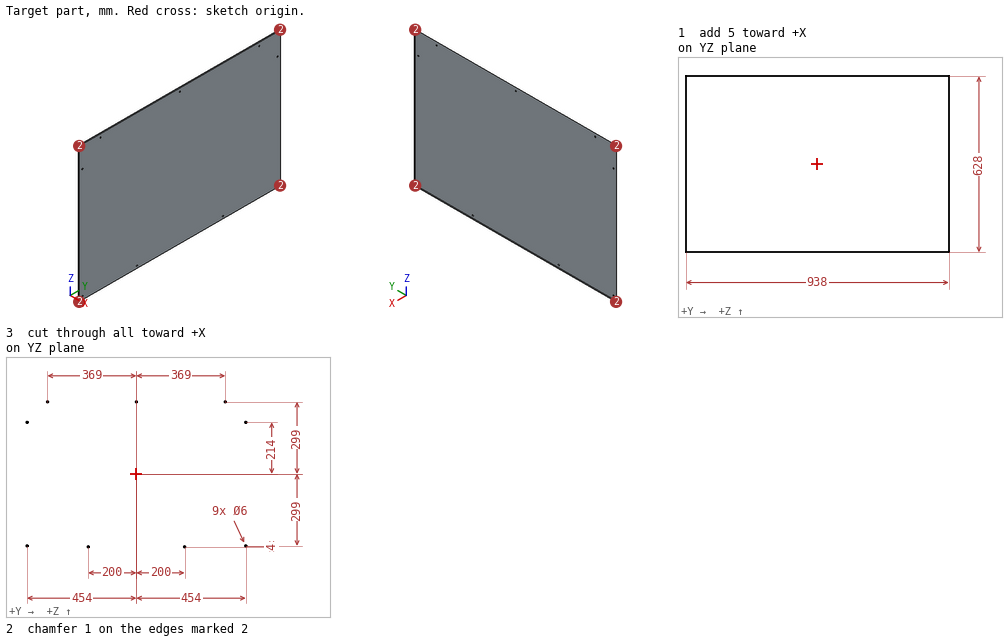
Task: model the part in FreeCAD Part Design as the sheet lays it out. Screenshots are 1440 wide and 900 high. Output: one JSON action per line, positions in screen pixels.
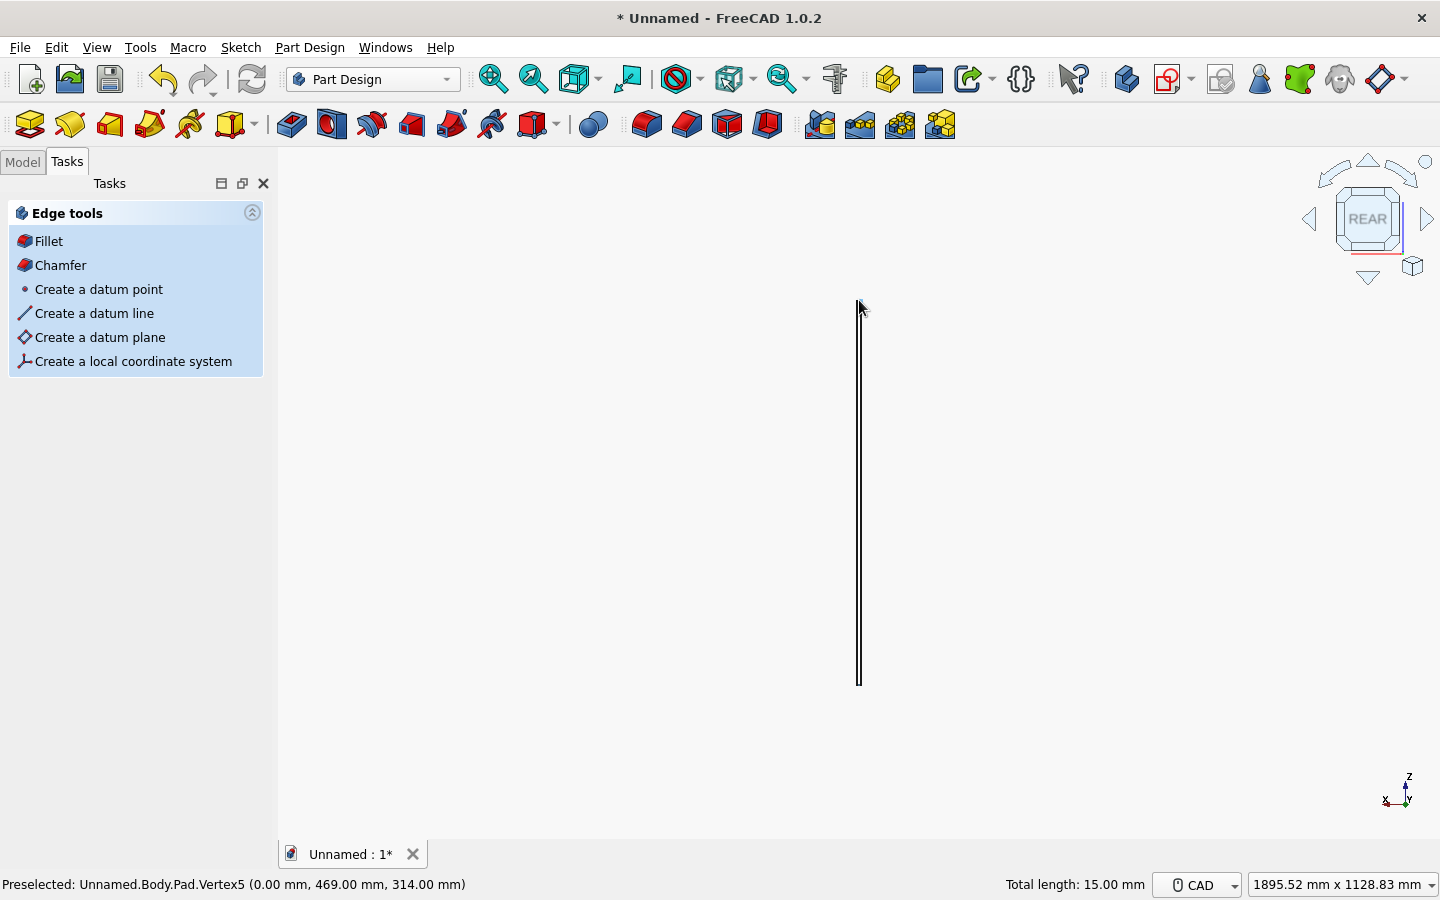
{"action": "key", "text": "6"}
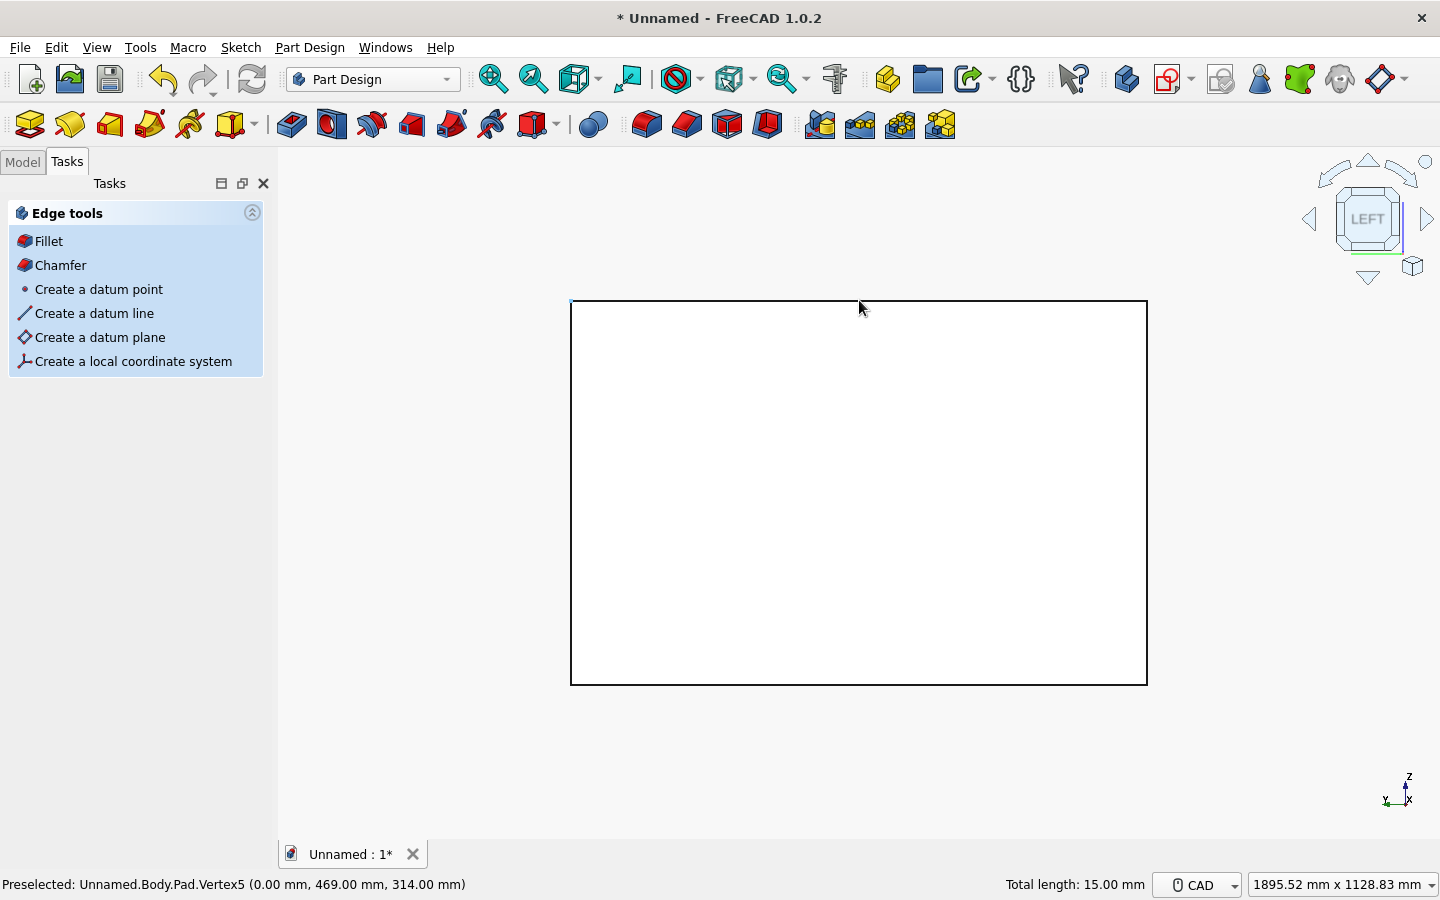
{"action": "scroll", "coordinate": [1147, 300], "scroll_direction": "up", "scroll_amount": 13}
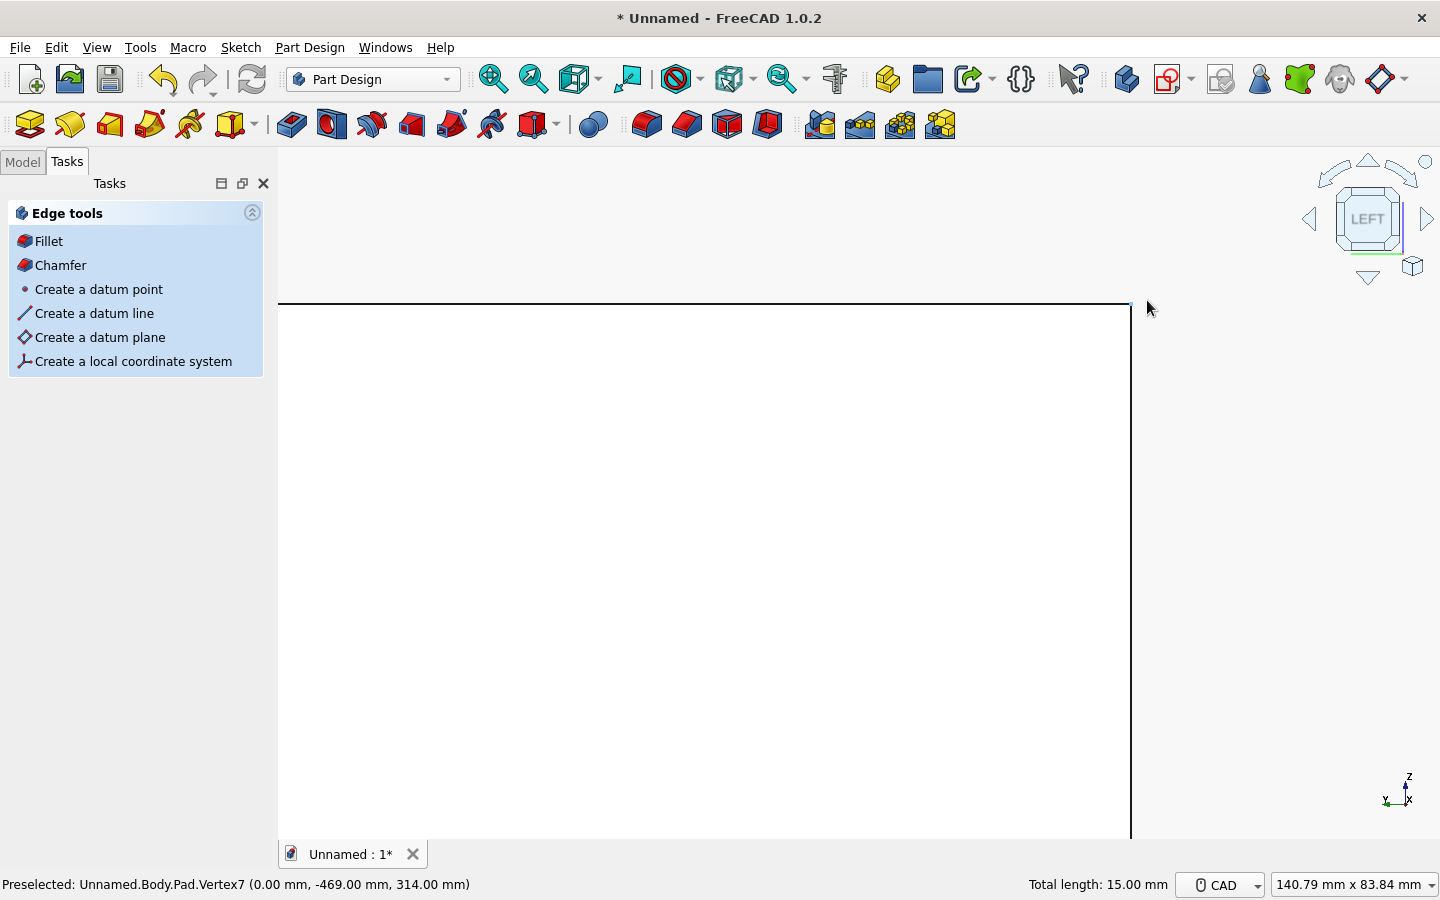
{"action": "key", "text": "v f"}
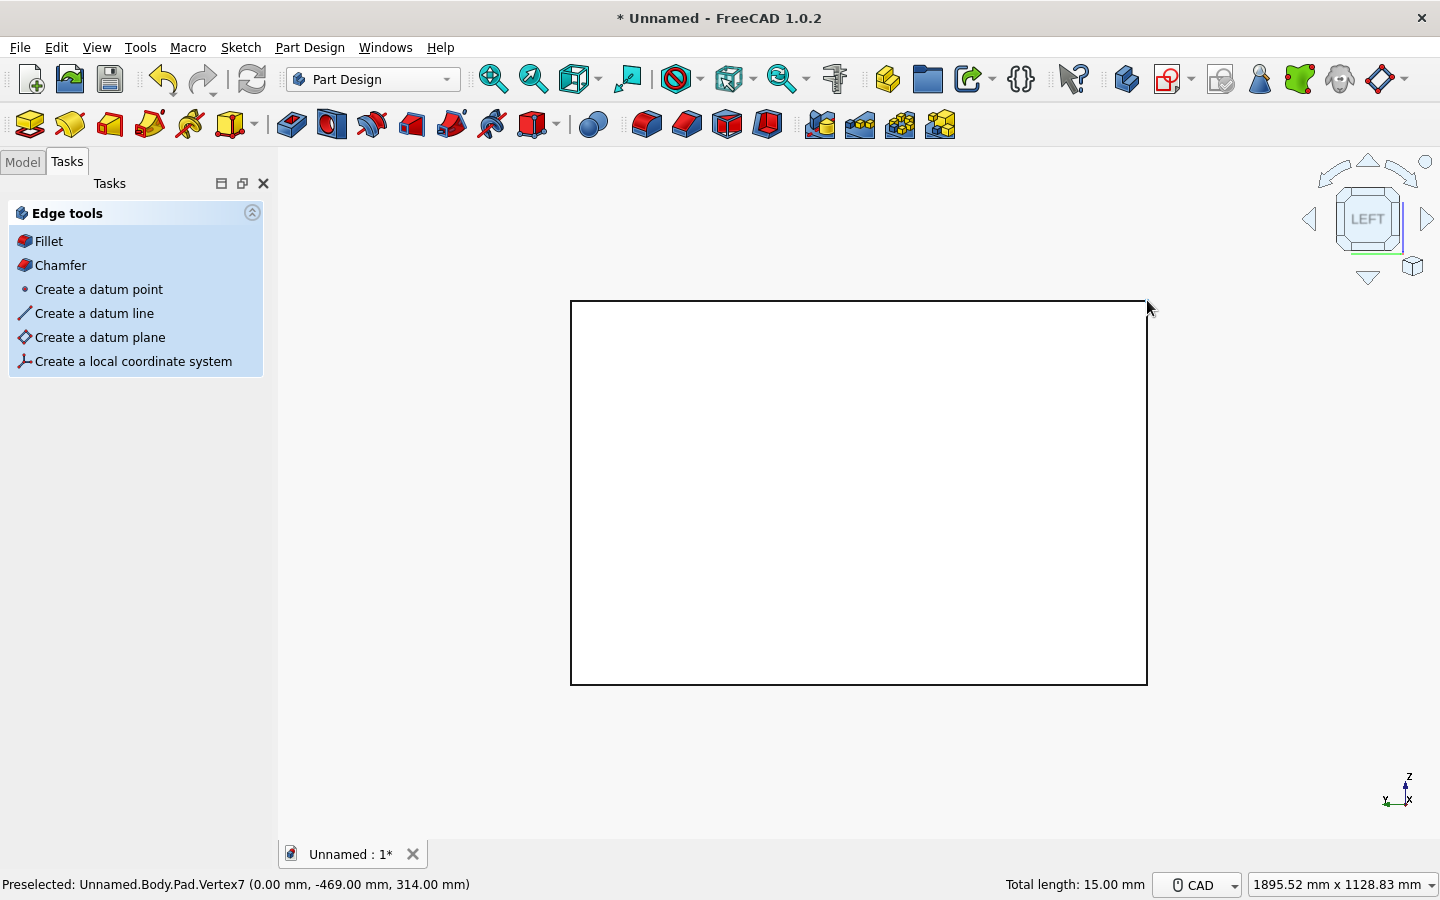
{"action": "key", "text": "v 3"}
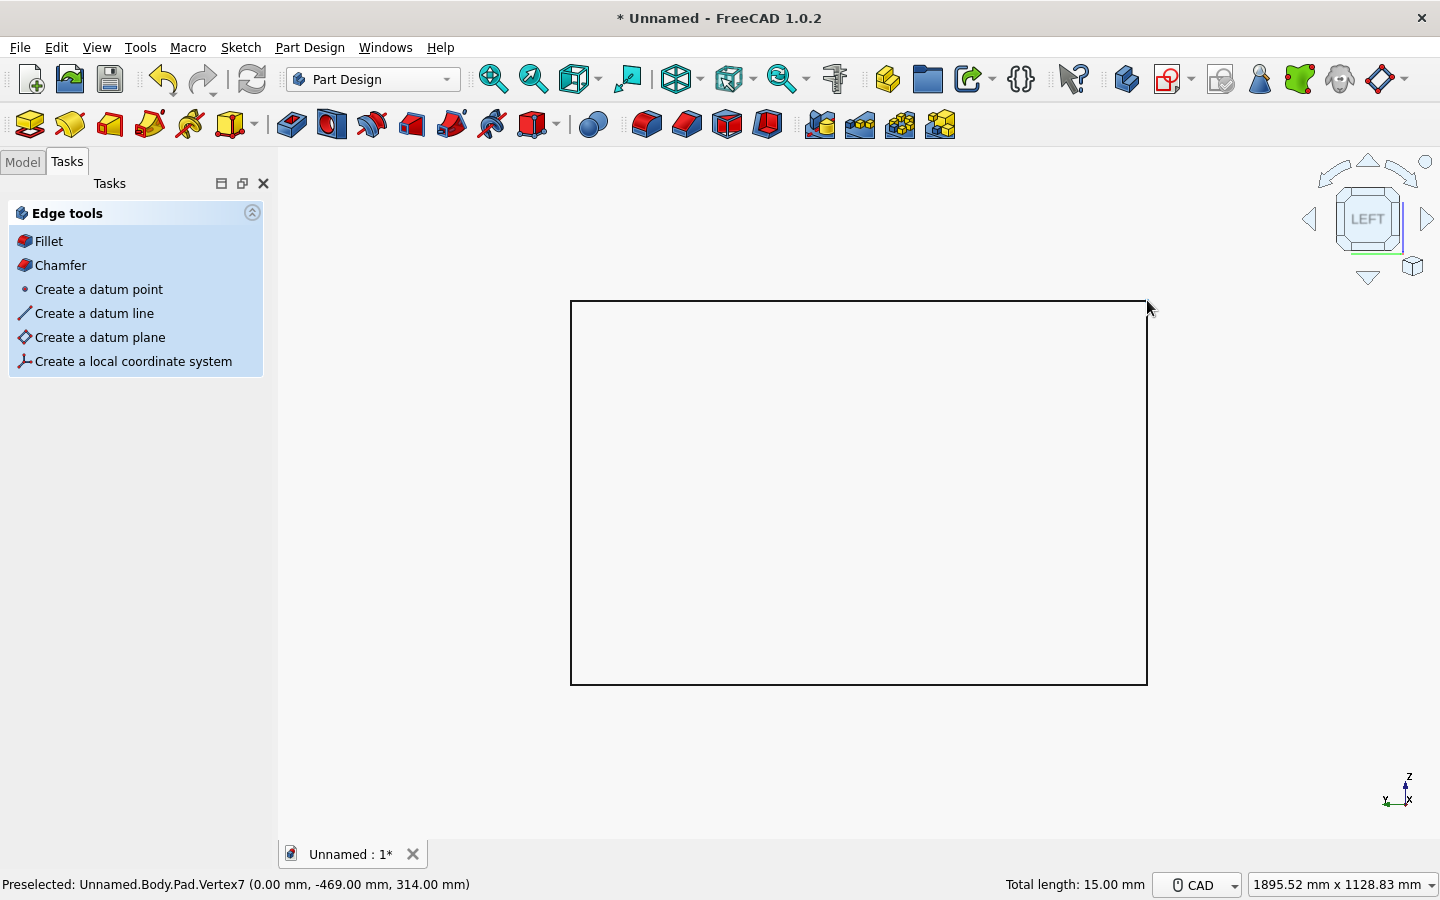
{"action": "key", "text": "0"}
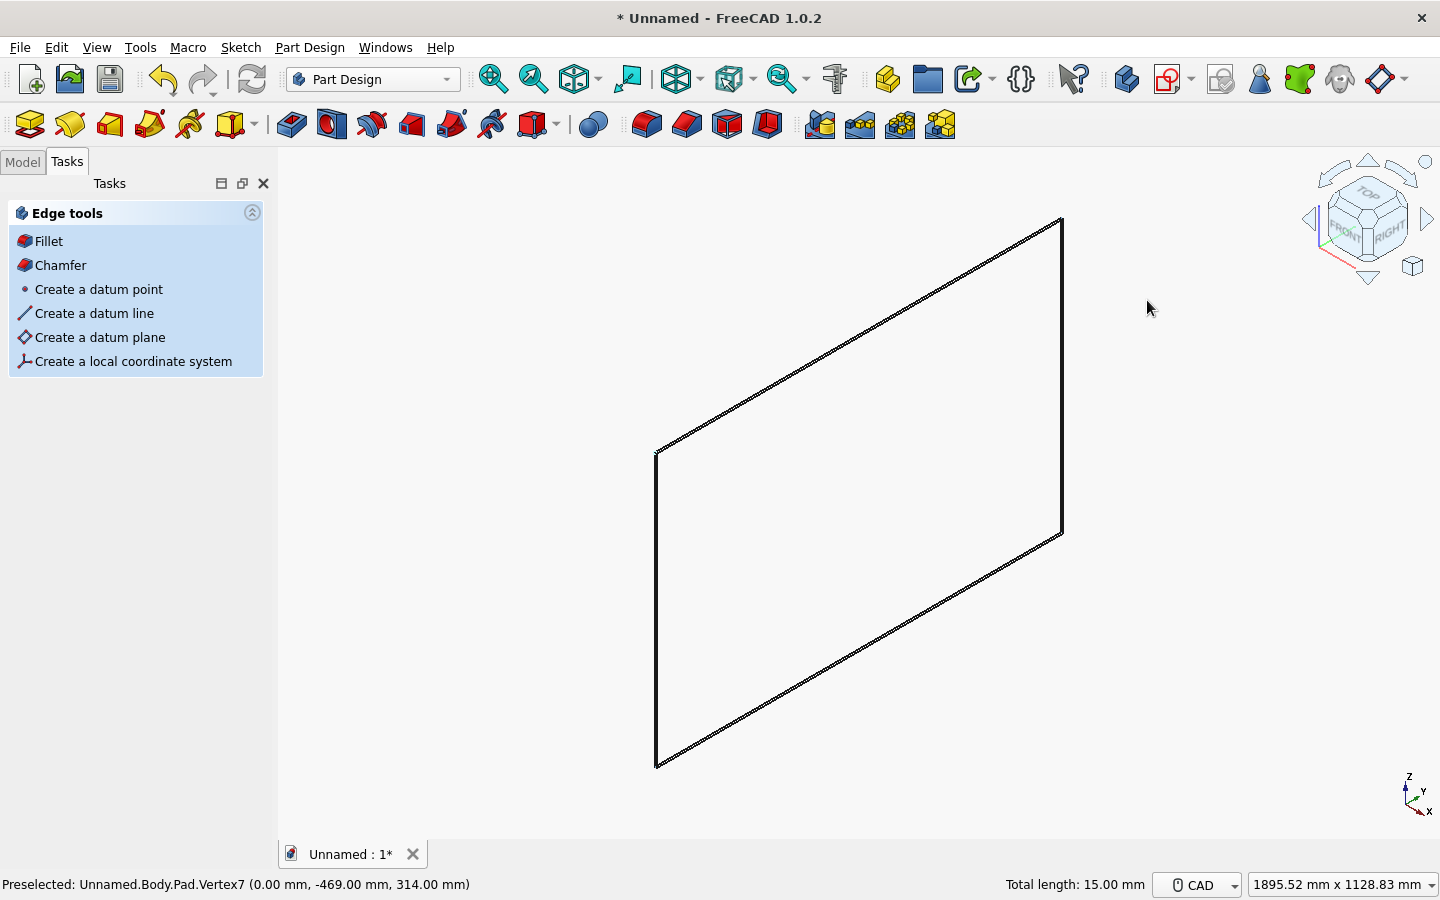
{"action": "scroll", "coordinate": [656, 452], "scroll_direction": "up", "scroll_amount": 13}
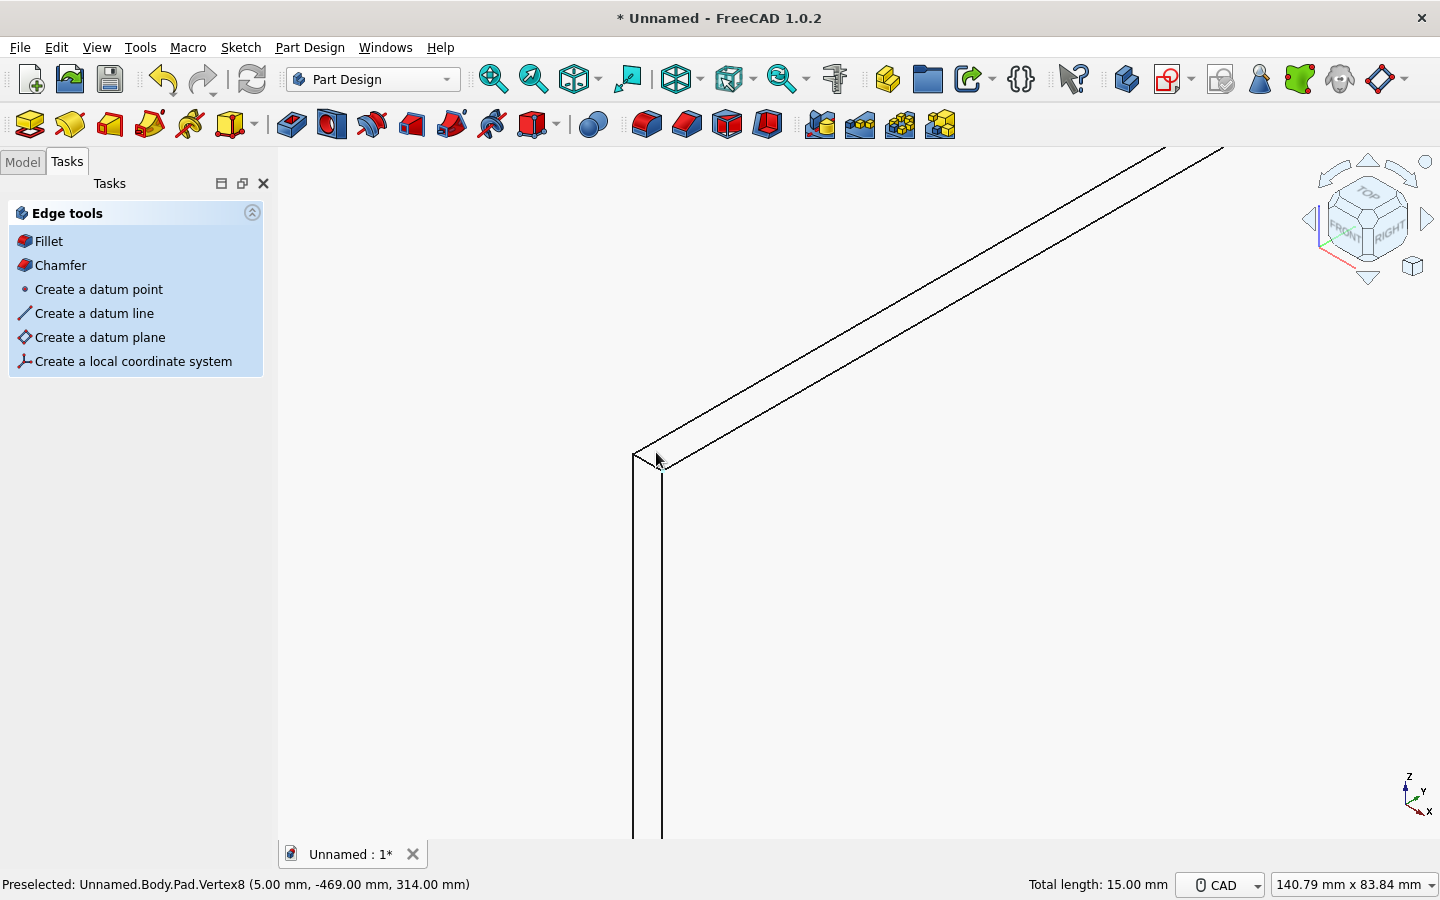
{"action": "left_click", "coordinate": [648, 462], "text": "ctrl"}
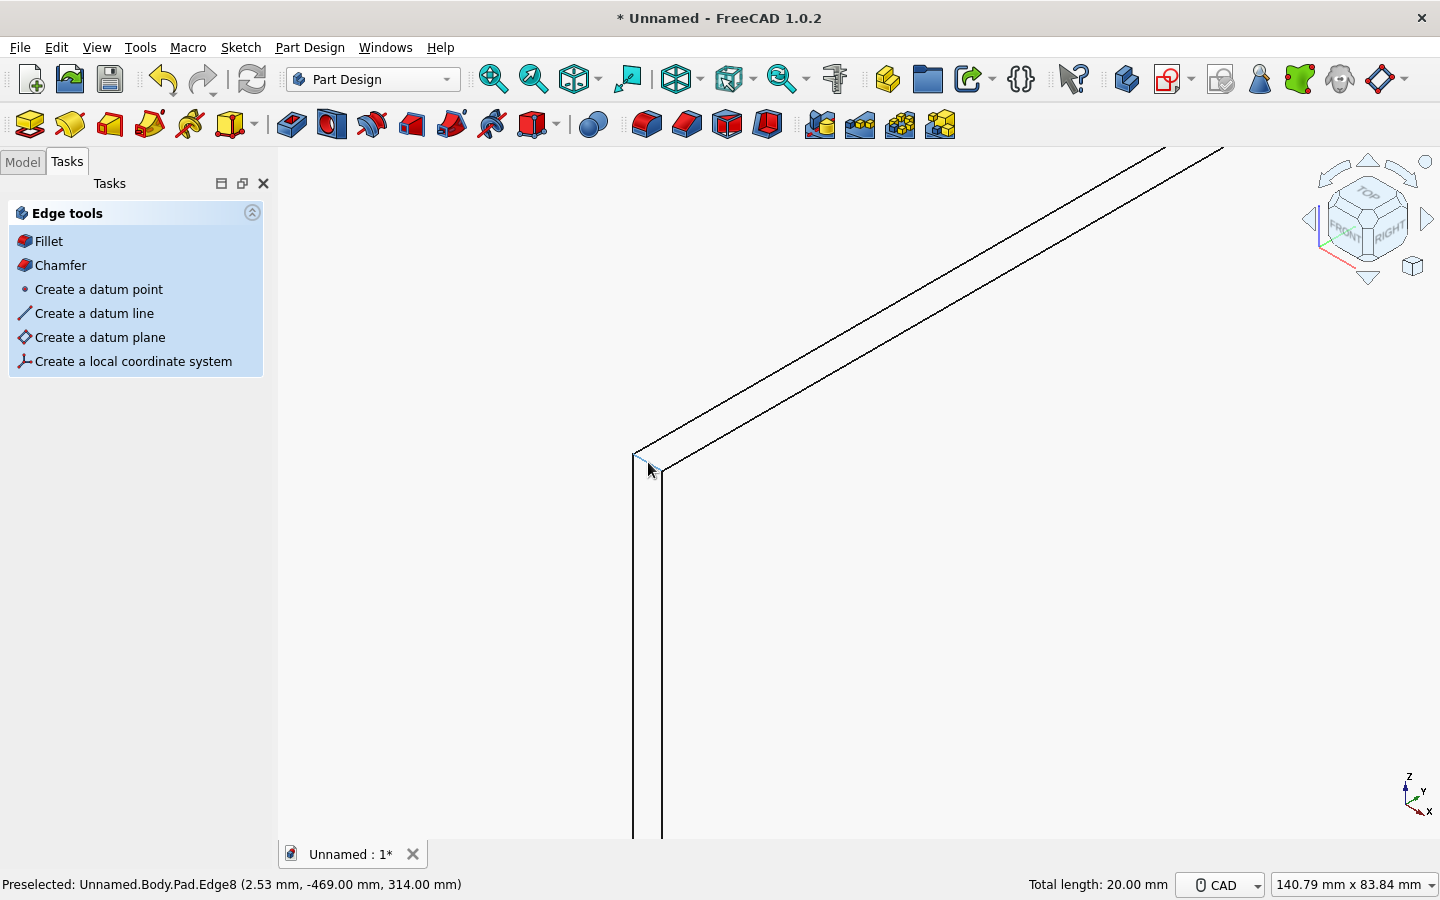
{"action": "key", "text": "v 1"}